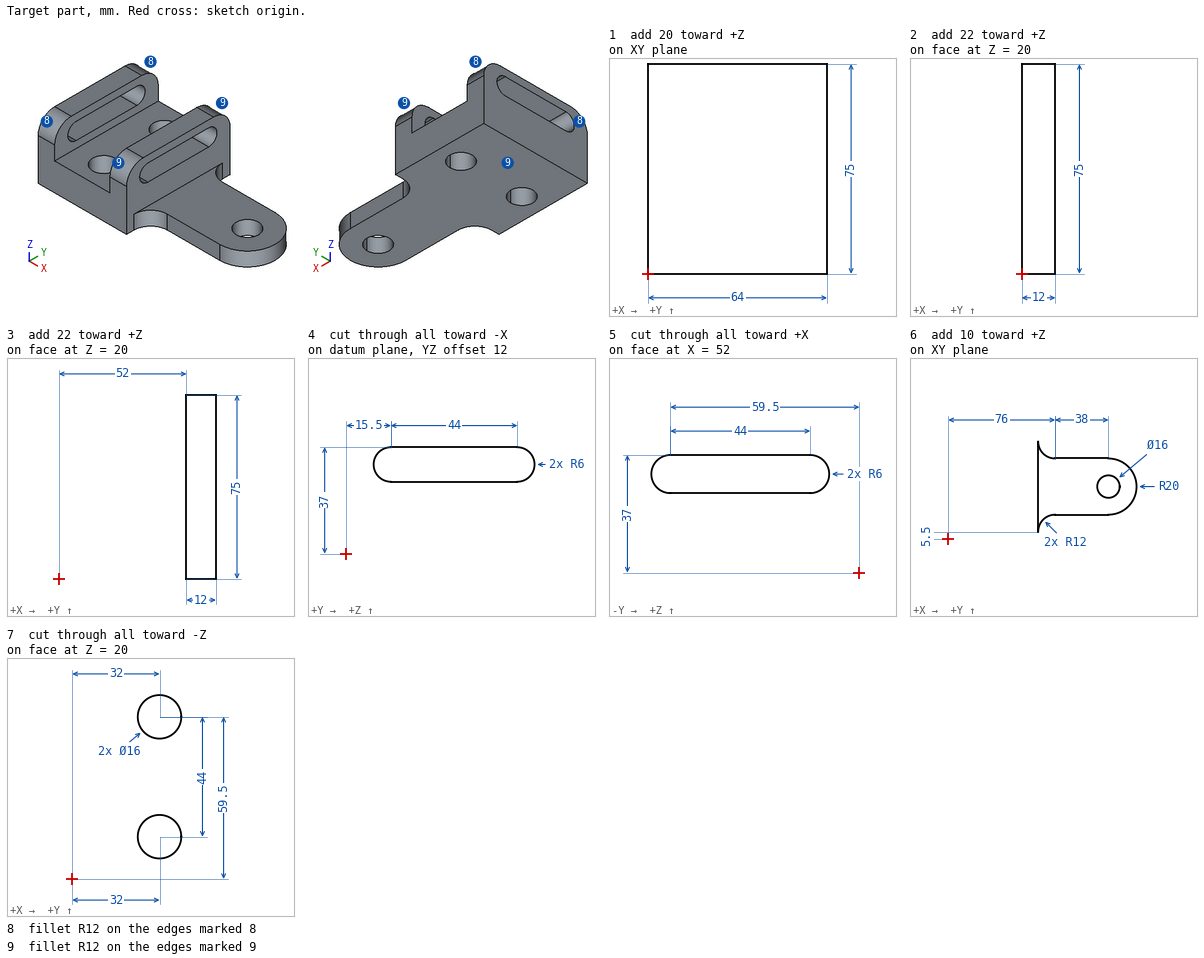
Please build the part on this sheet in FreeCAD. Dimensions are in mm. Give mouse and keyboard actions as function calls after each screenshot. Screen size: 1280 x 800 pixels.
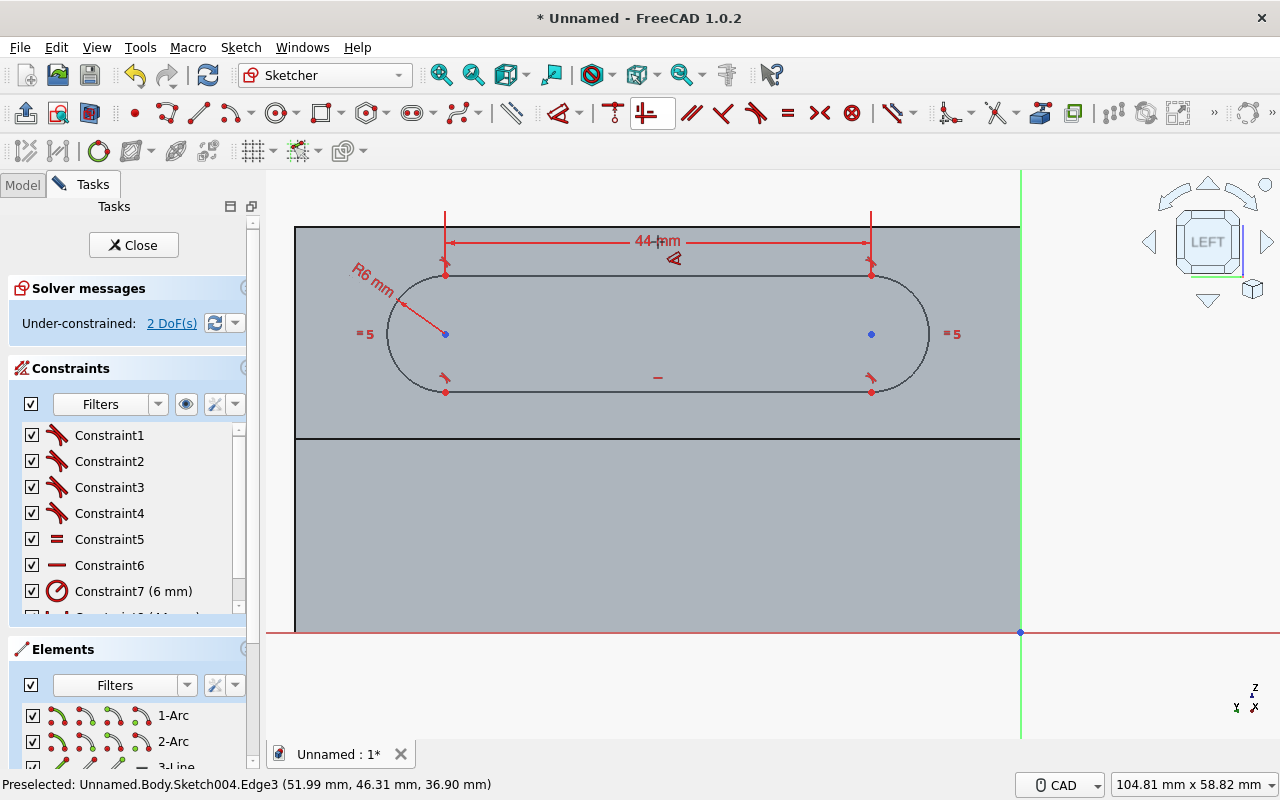
click(445, 276)
click(1055, 454)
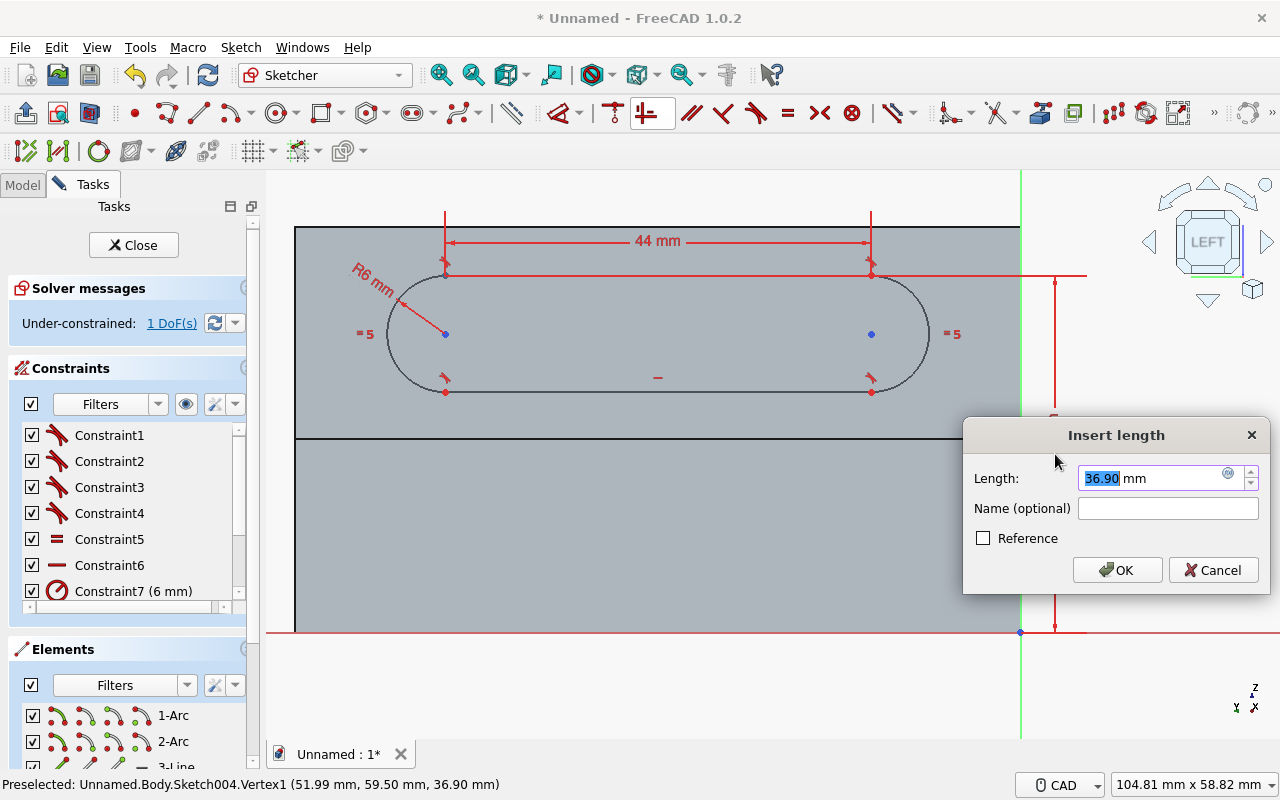
text(37)
key(Return)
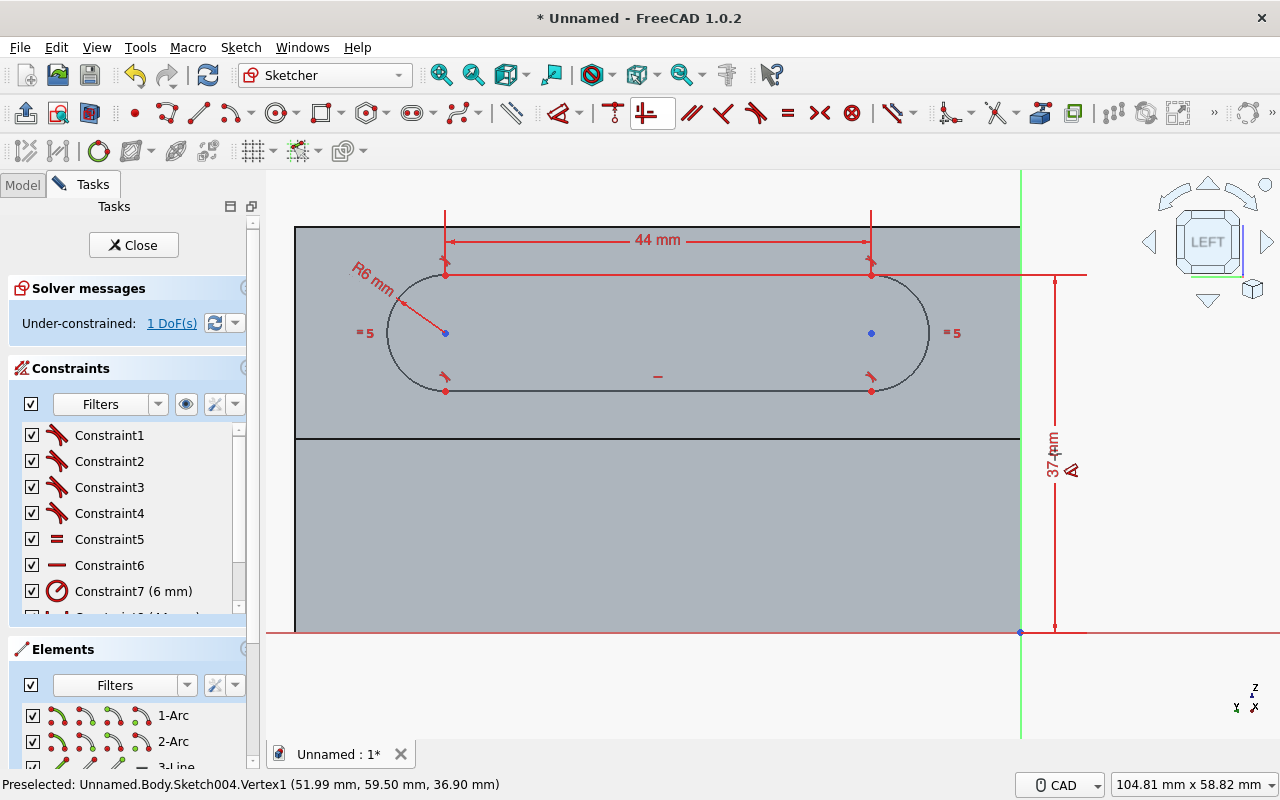
click(445, 275)
click(733, 667)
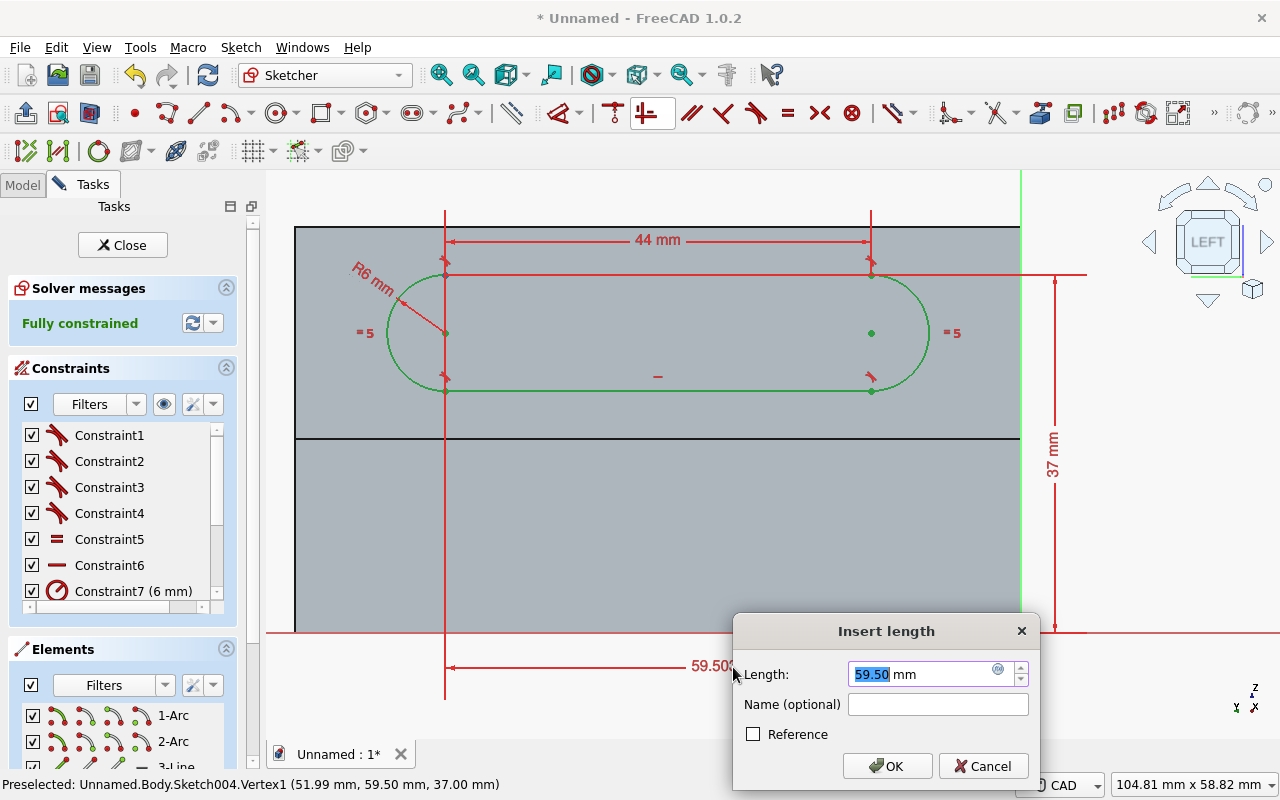
text(59.5)
key(Return)
key(Escape)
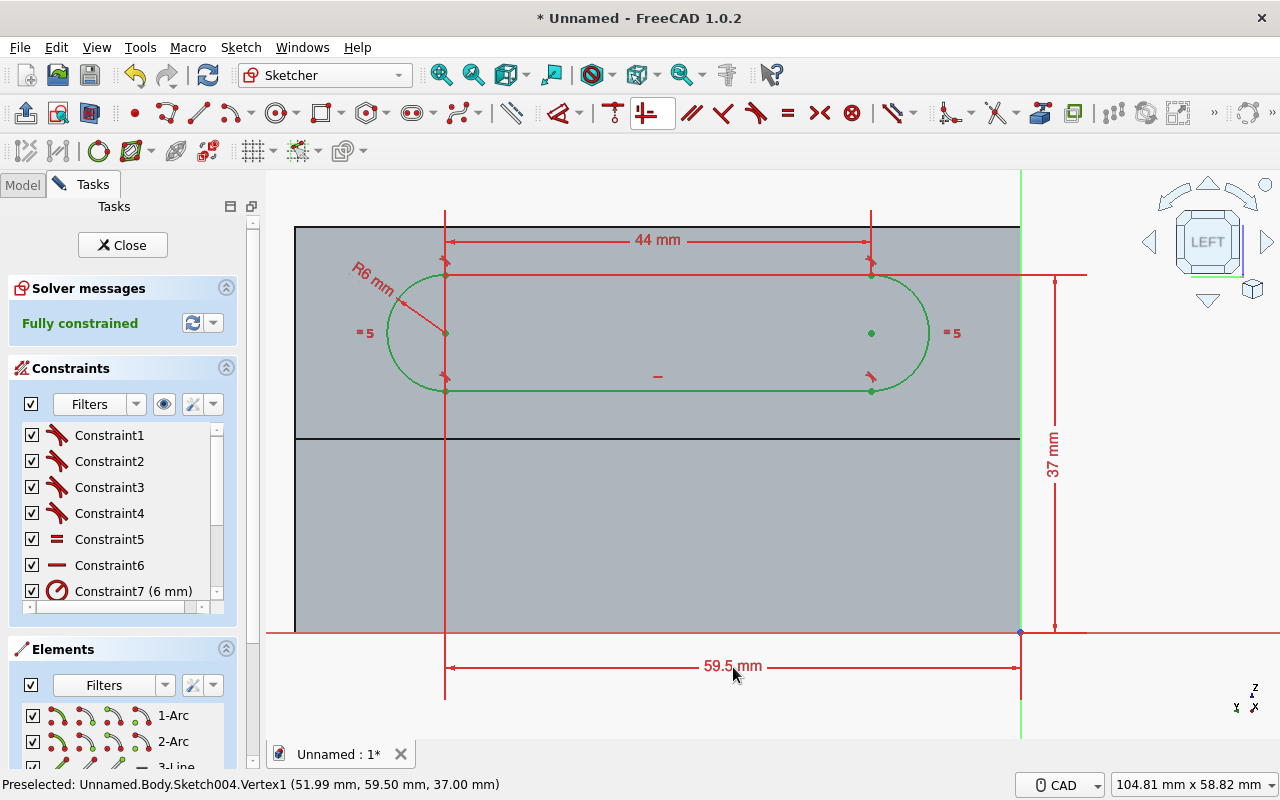
click(123, 245)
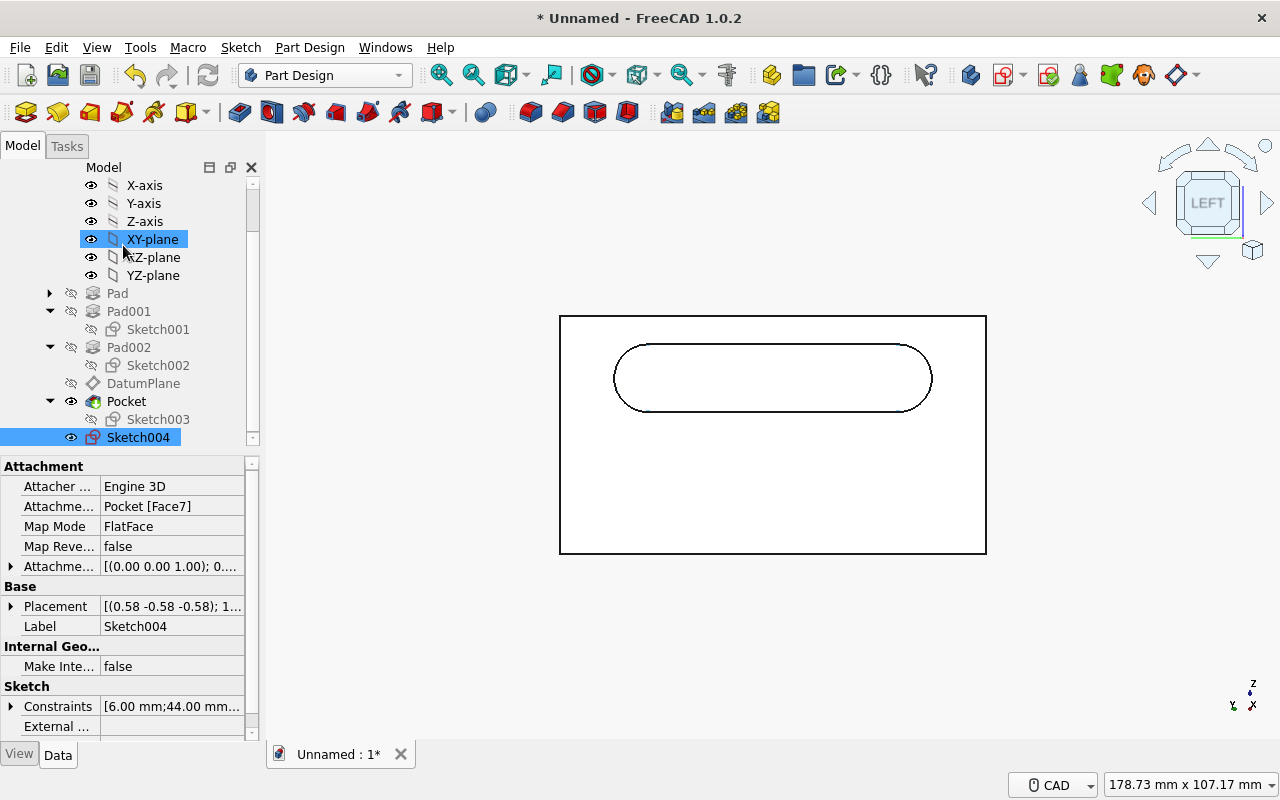
click(240, 112)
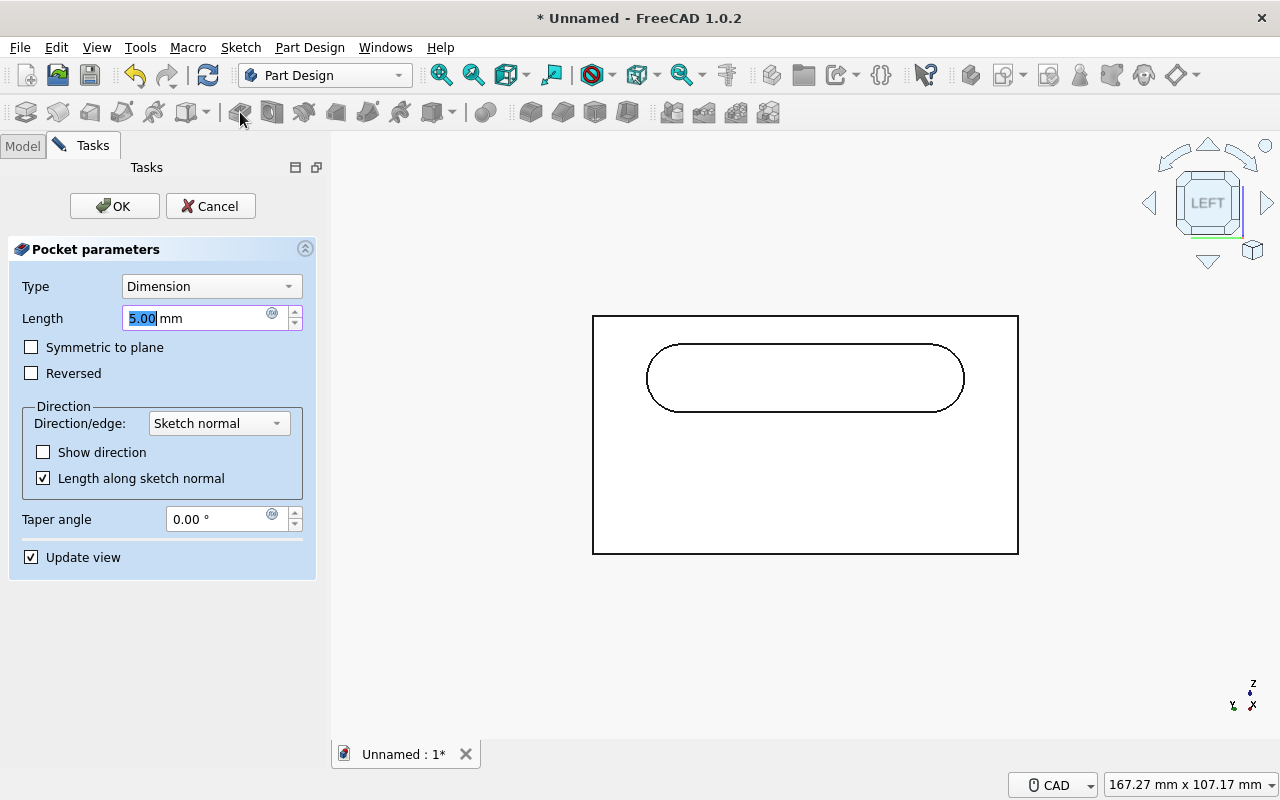
click(212, 286)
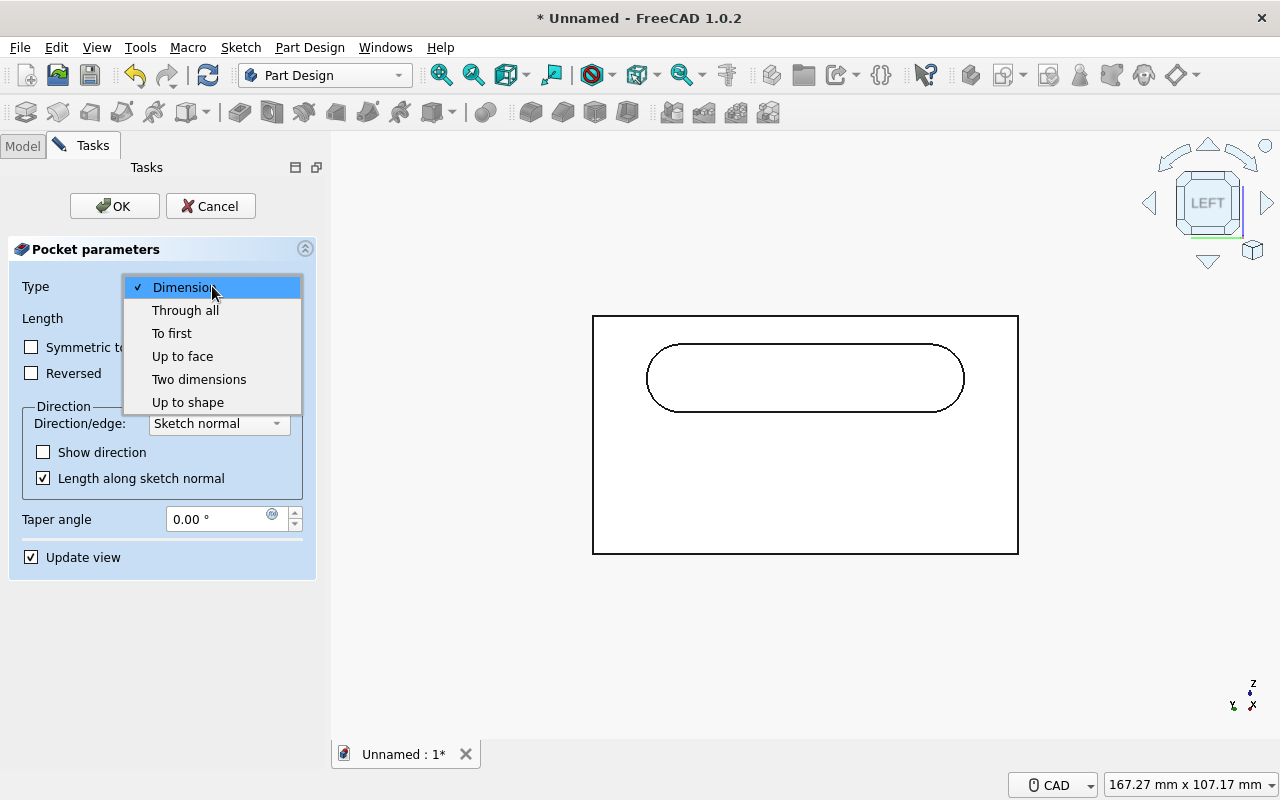
click(212, 310)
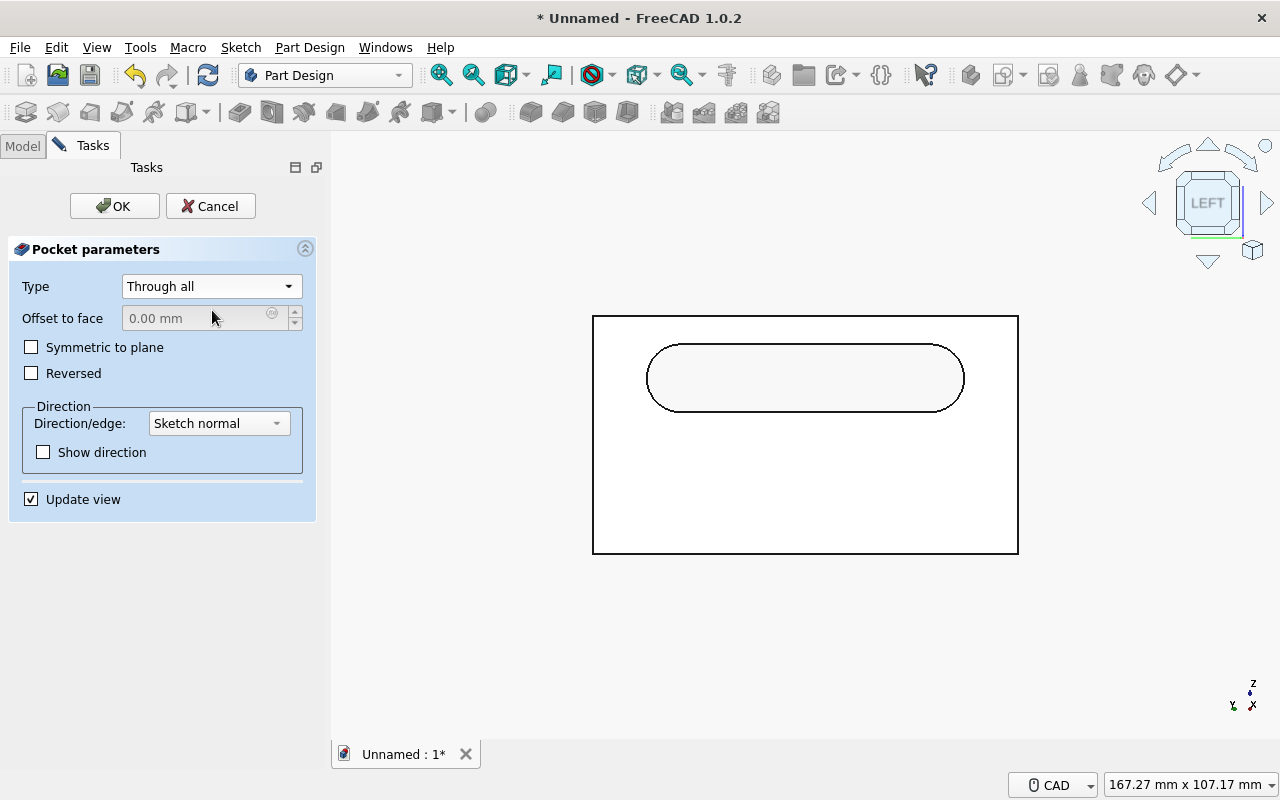
click(115, 206)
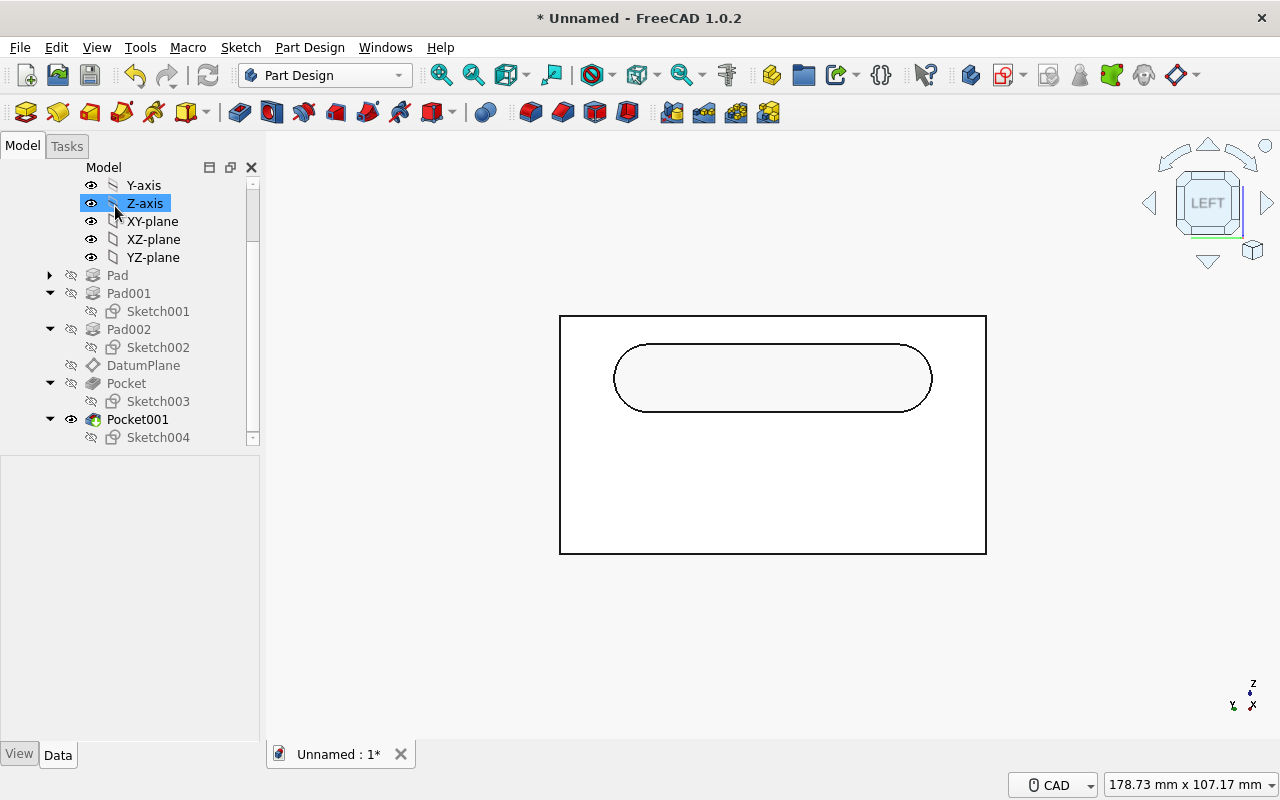
click(442, 76)